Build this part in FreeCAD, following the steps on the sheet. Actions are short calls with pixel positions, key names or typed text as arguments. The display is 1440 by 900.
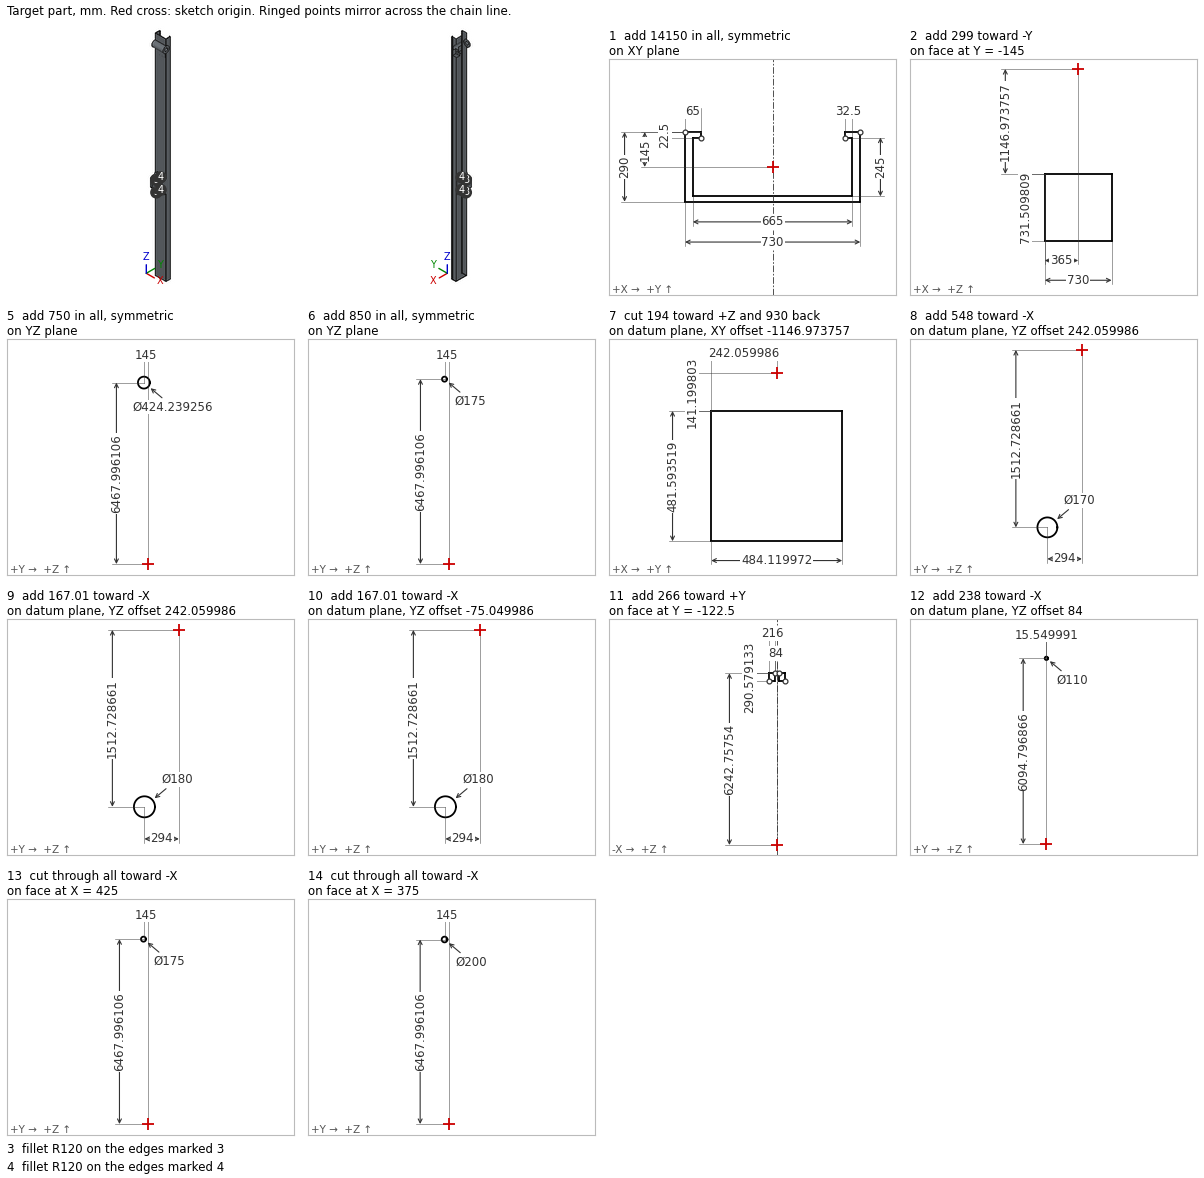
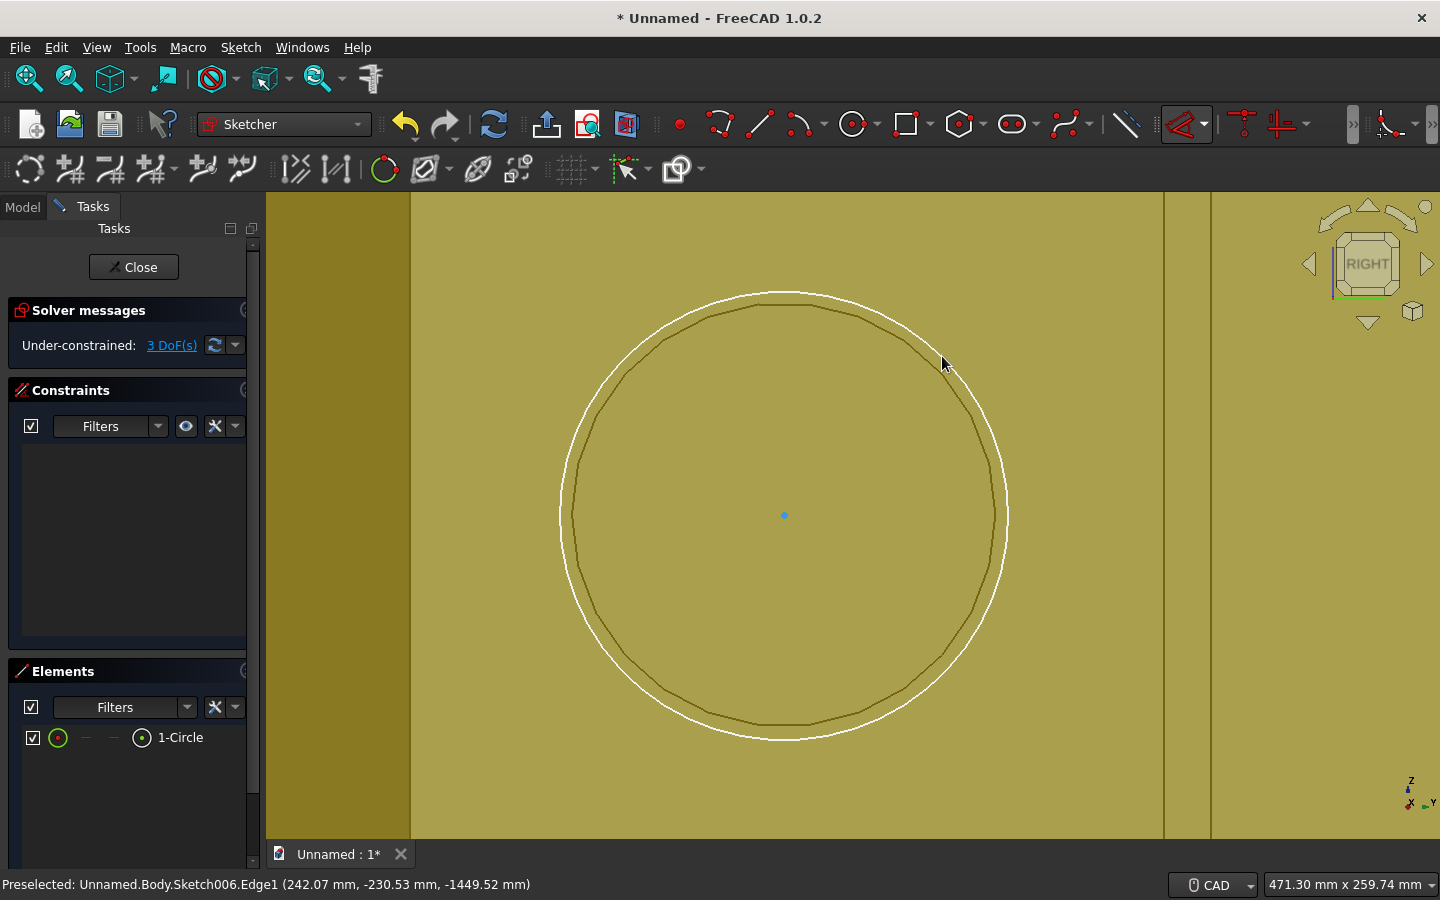
click(942, 357)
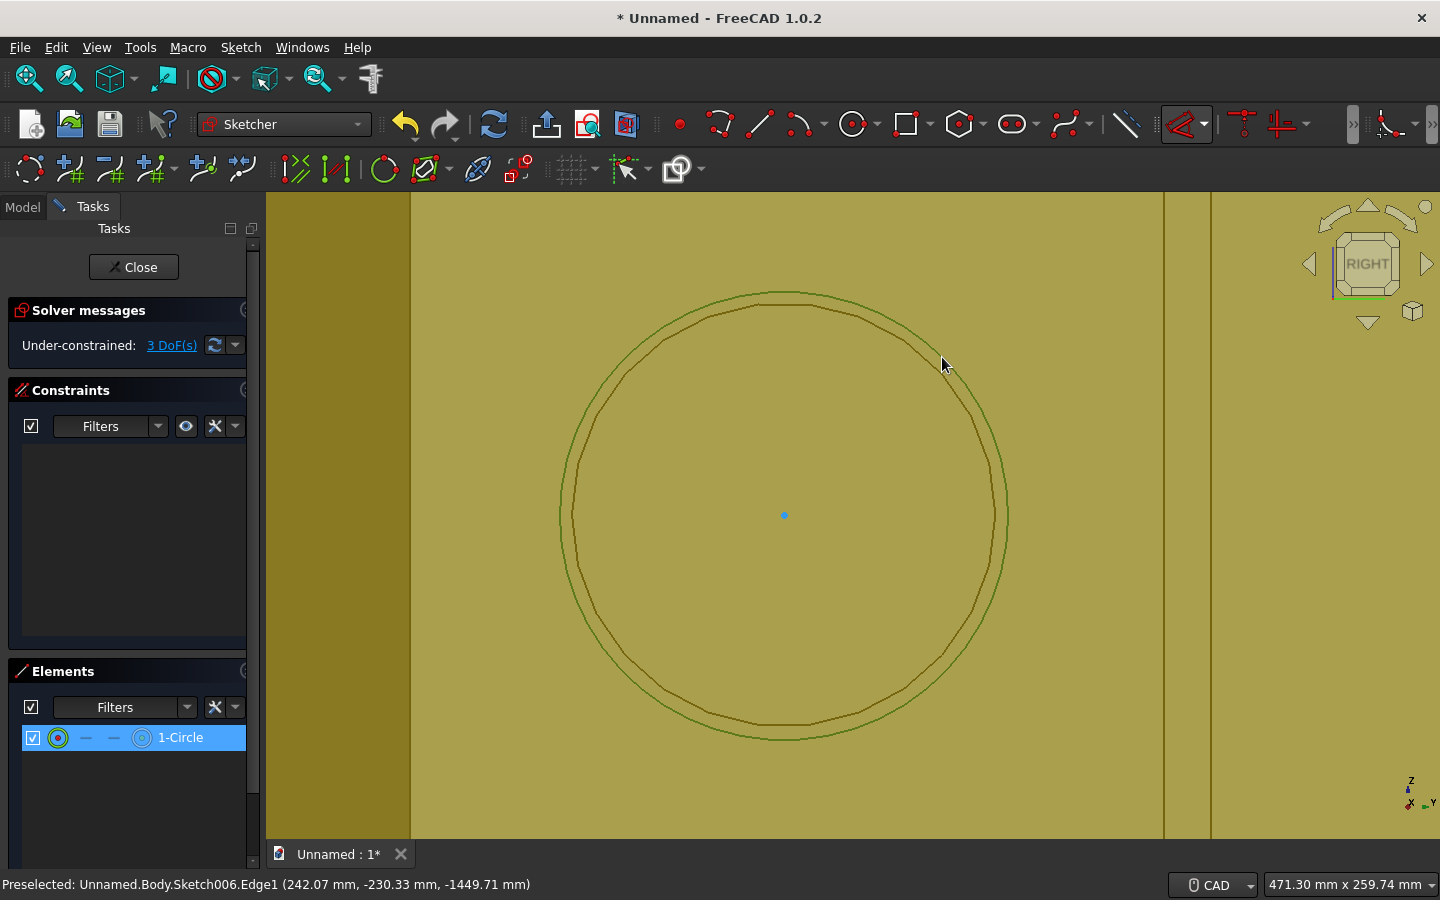
key(k)
key(o)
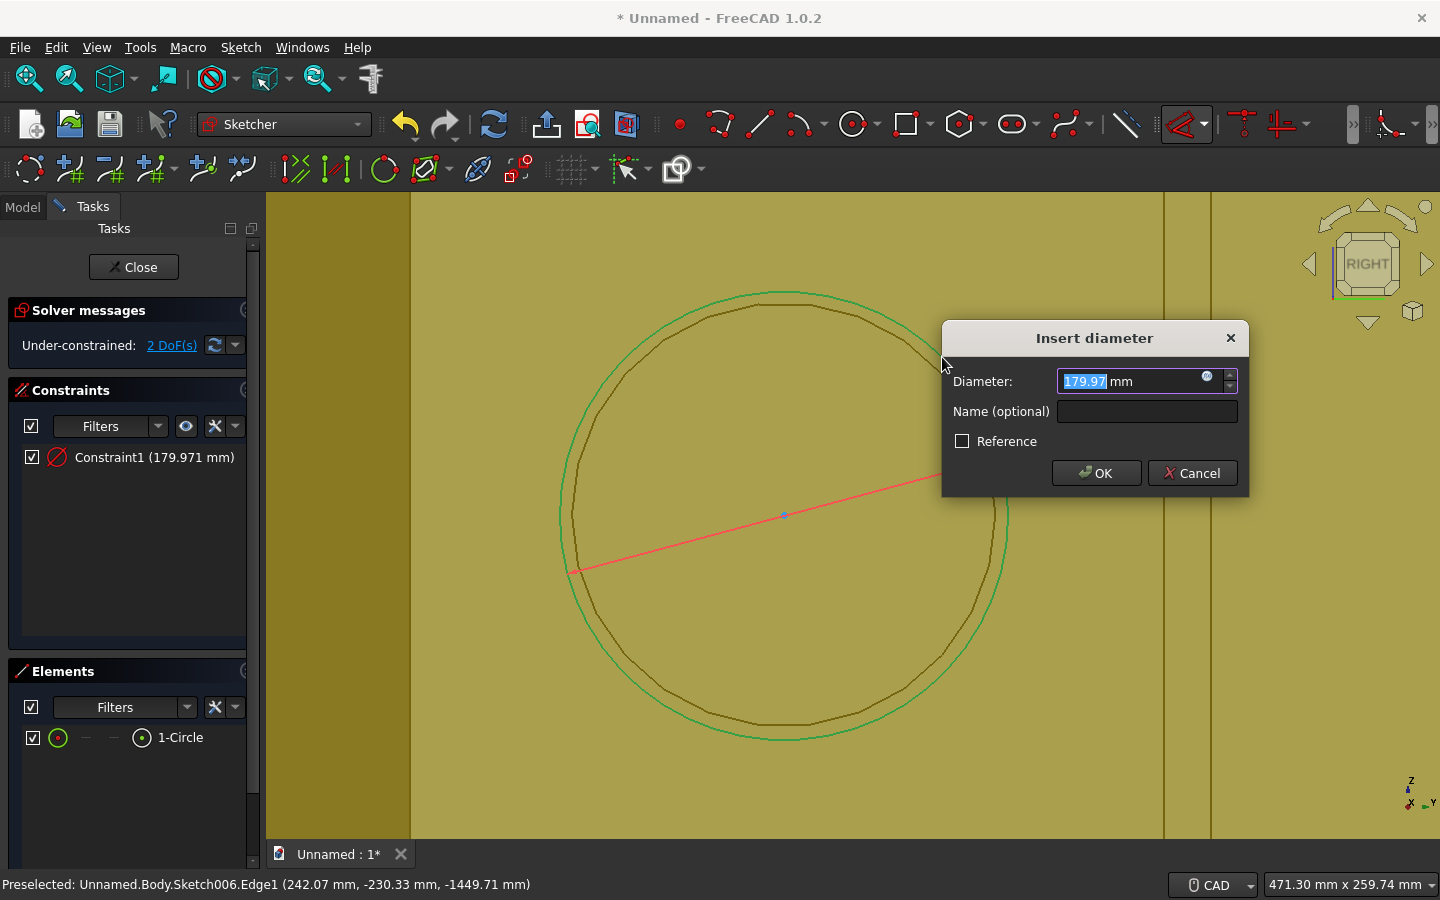
text(180)
key(Return)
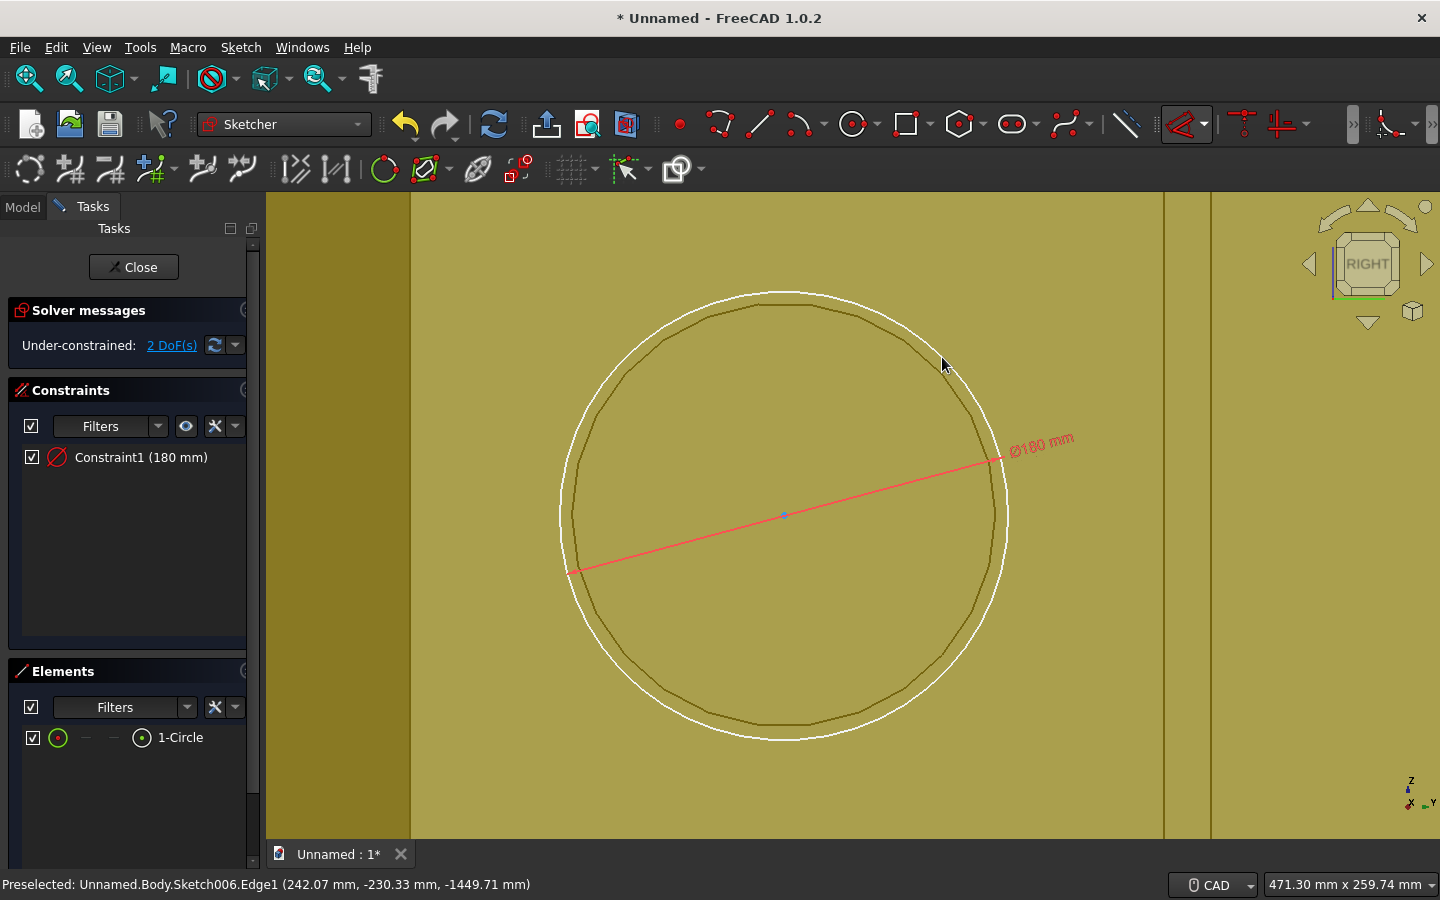
click(784, 516)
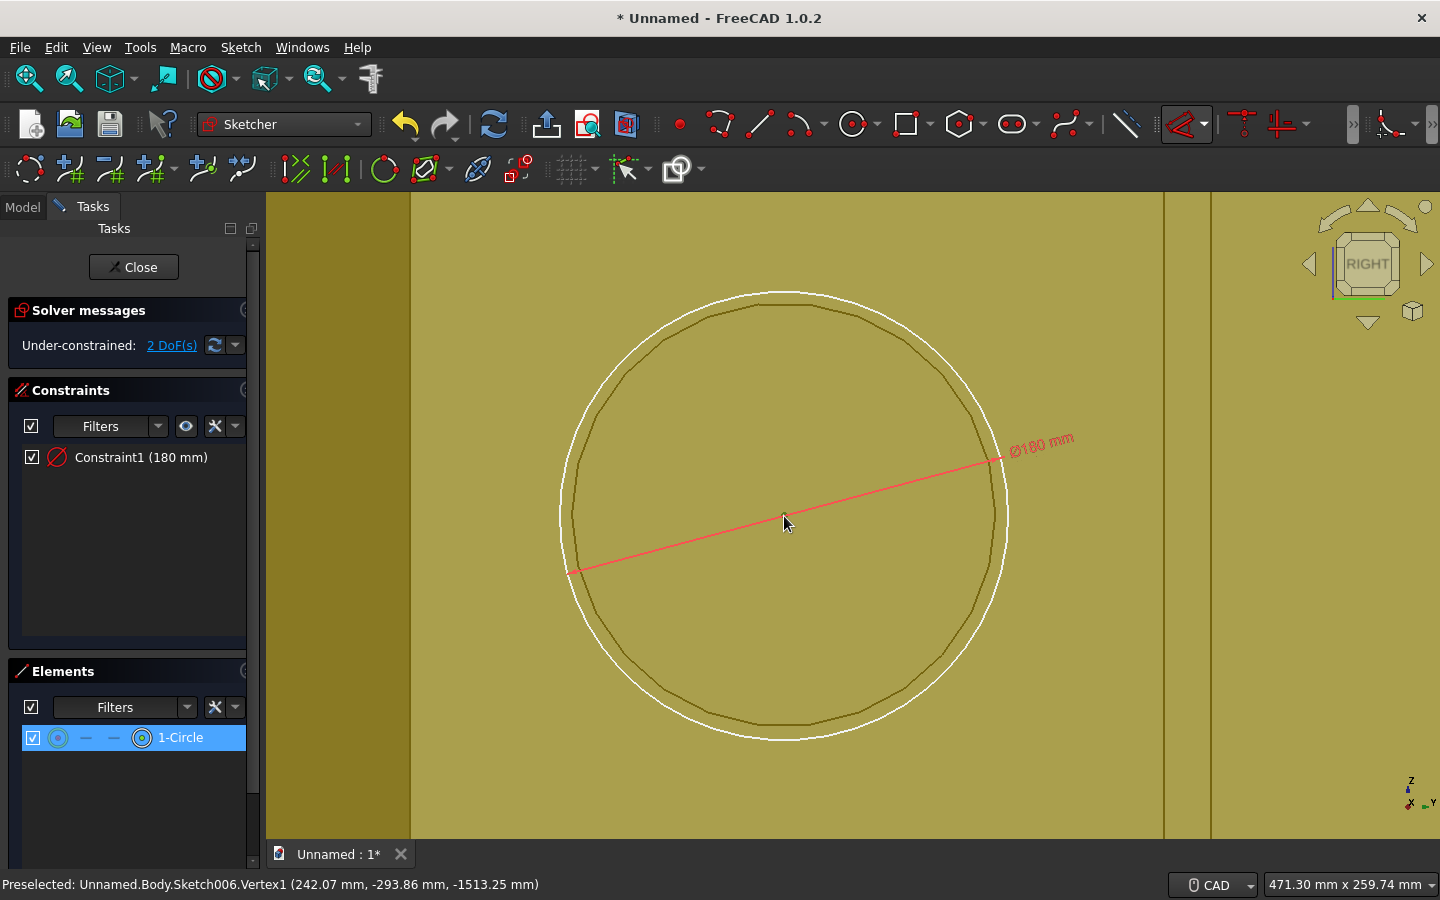
click(1206, 124)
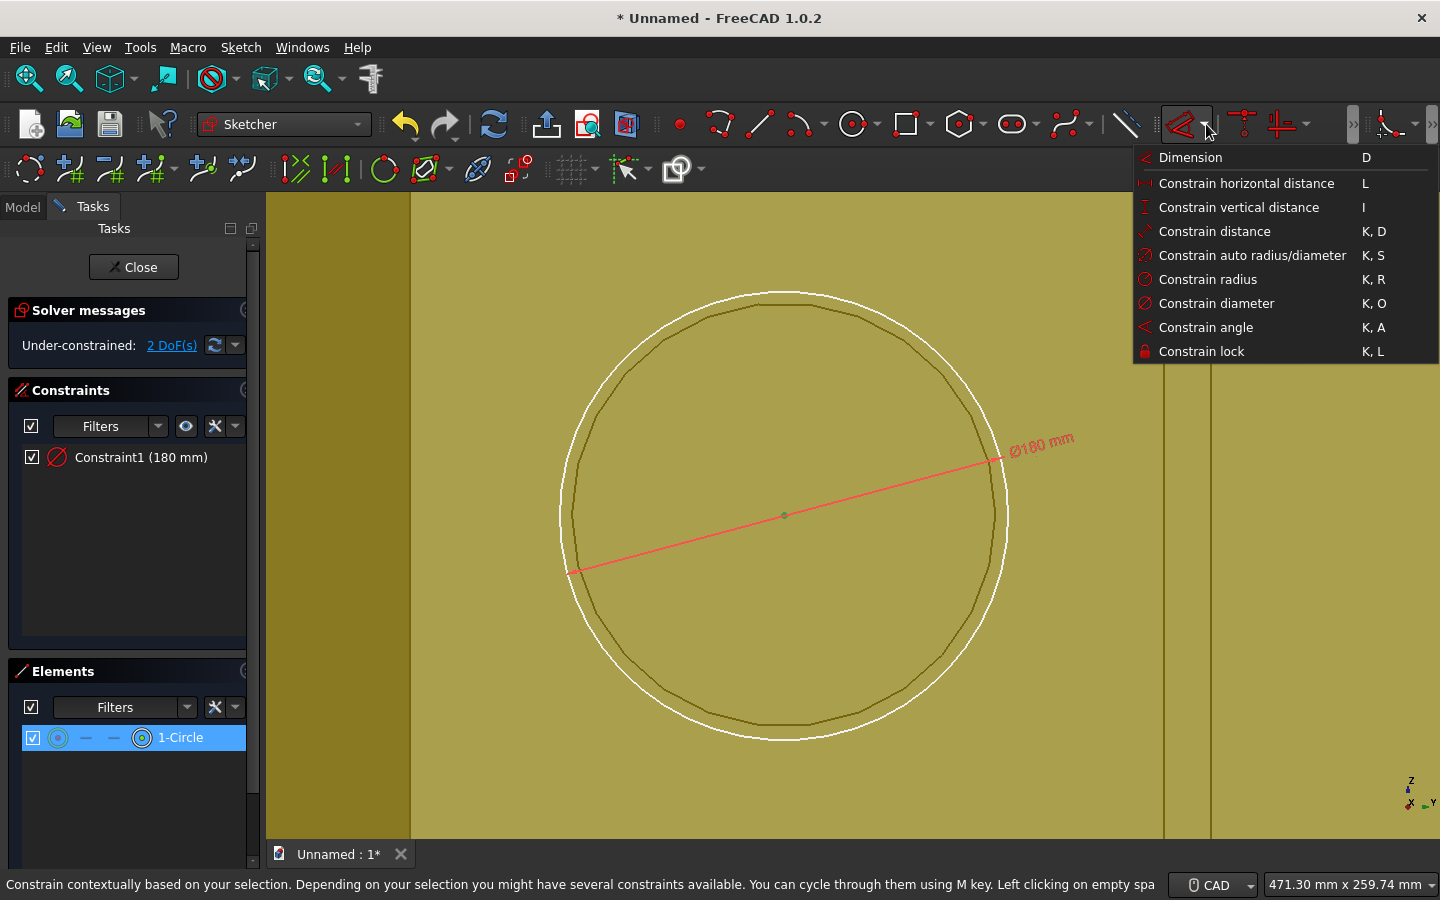
click(1286, 183)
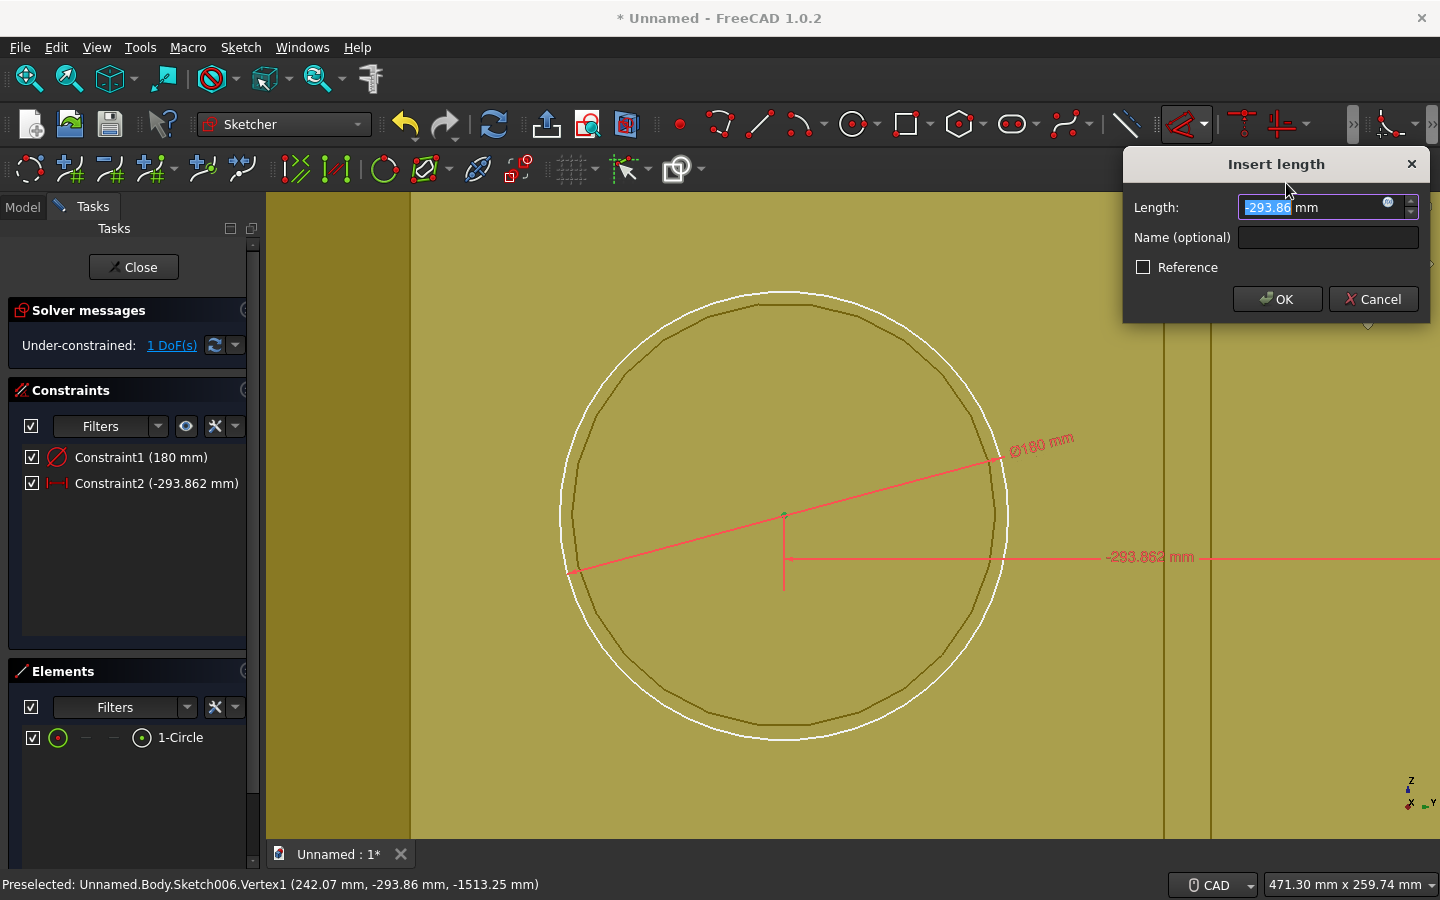
text(-294)
key(Return)